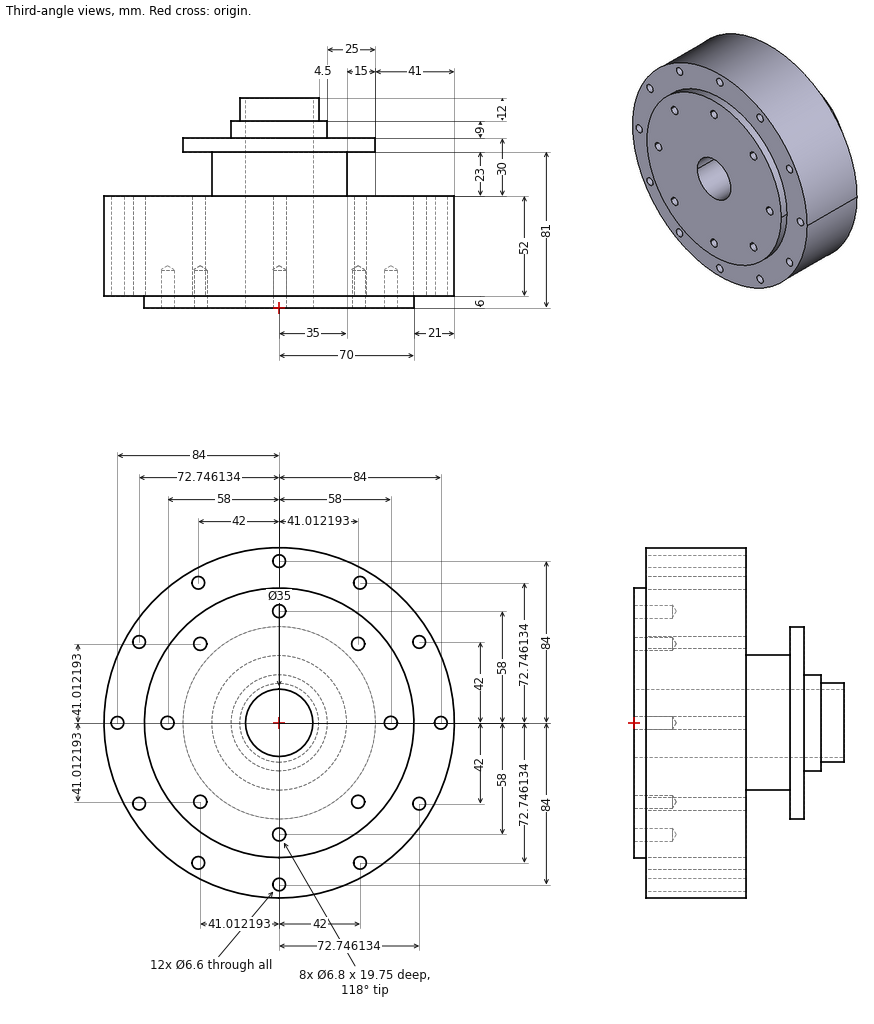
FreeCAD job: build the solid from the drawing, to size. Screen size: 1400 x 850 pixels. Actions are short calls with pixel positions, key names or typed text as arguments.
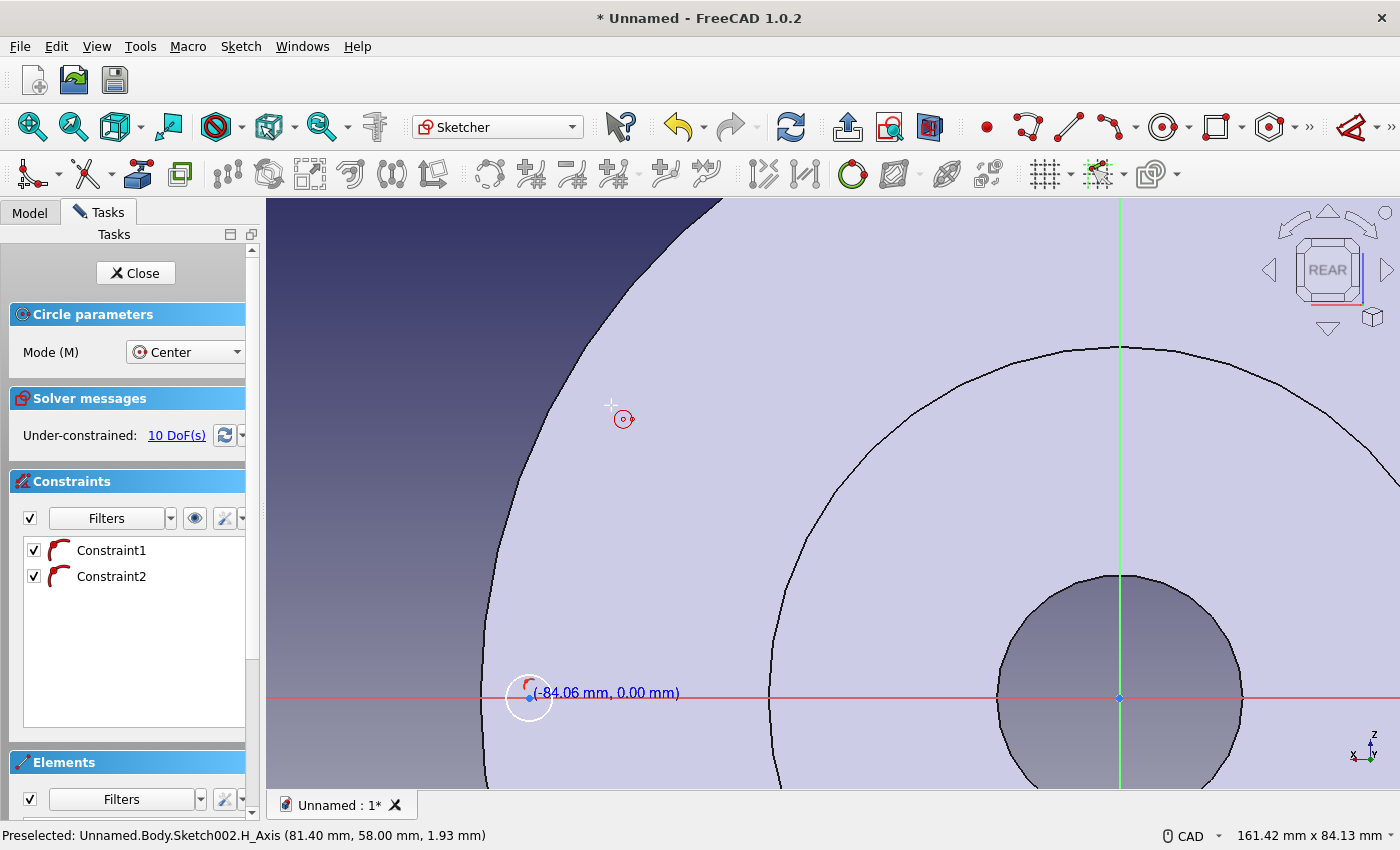
click(609, 403)
click(625, 387)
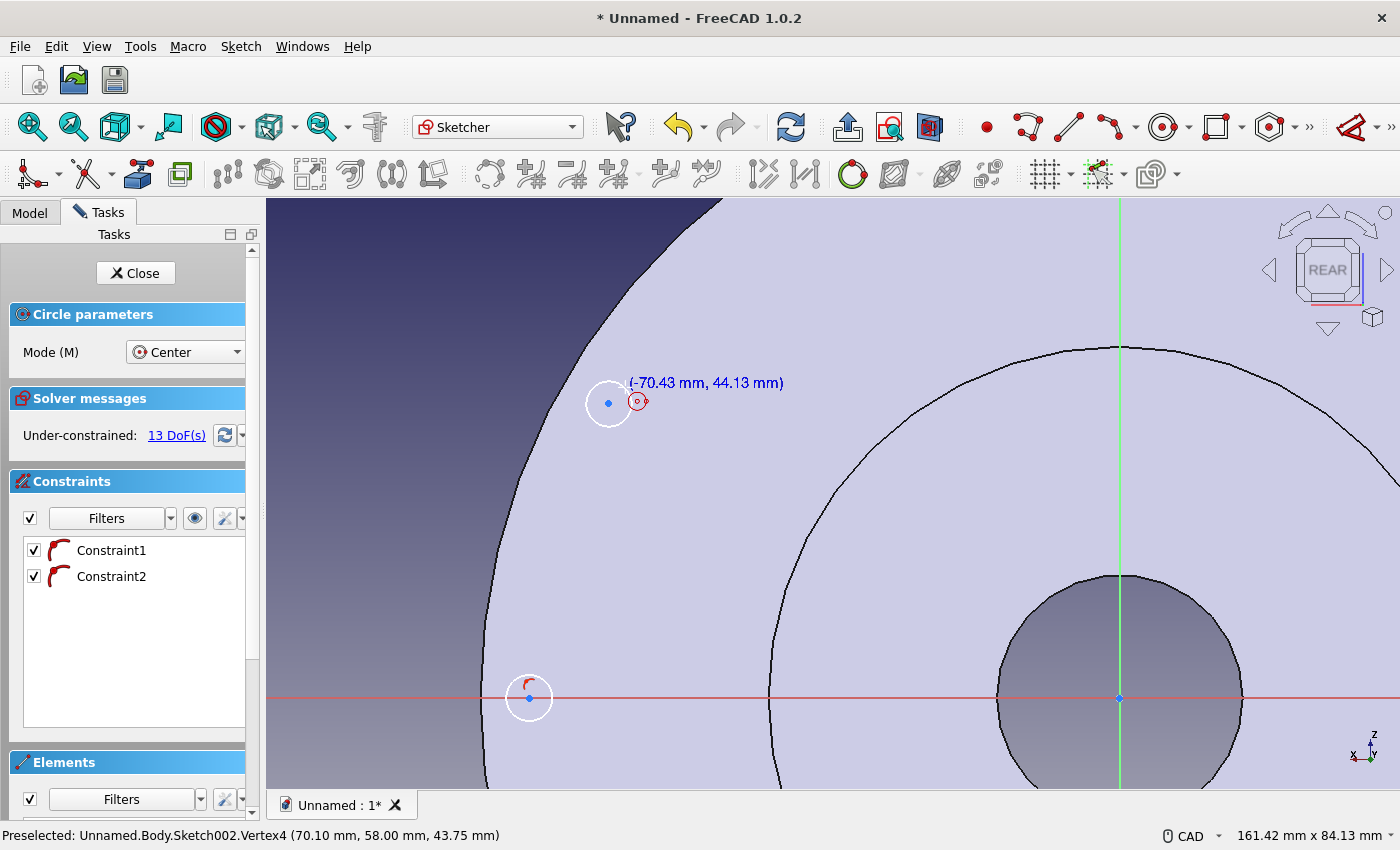
scroll(611, 405, down, 6)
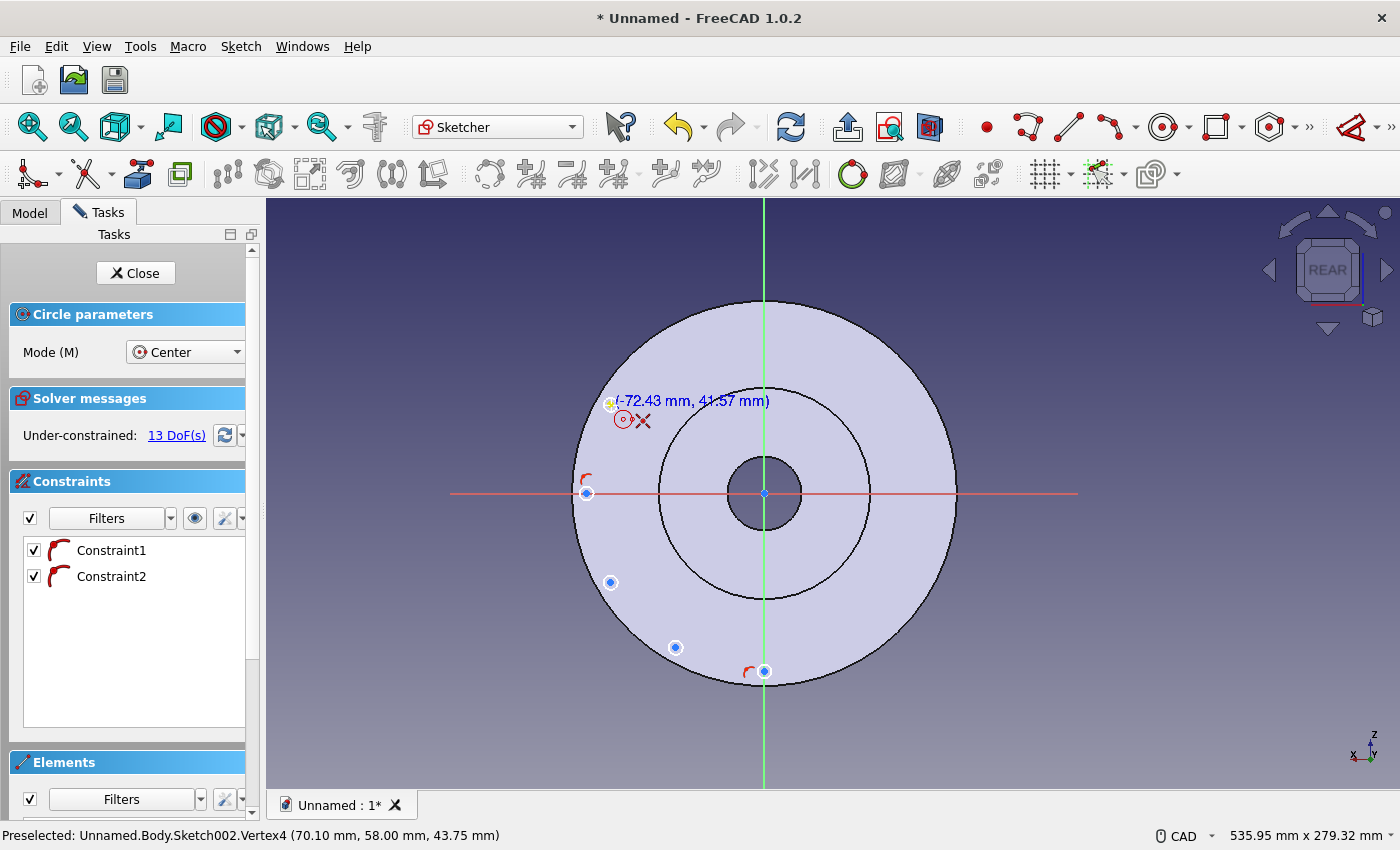
scroll(676, 340, up, 6)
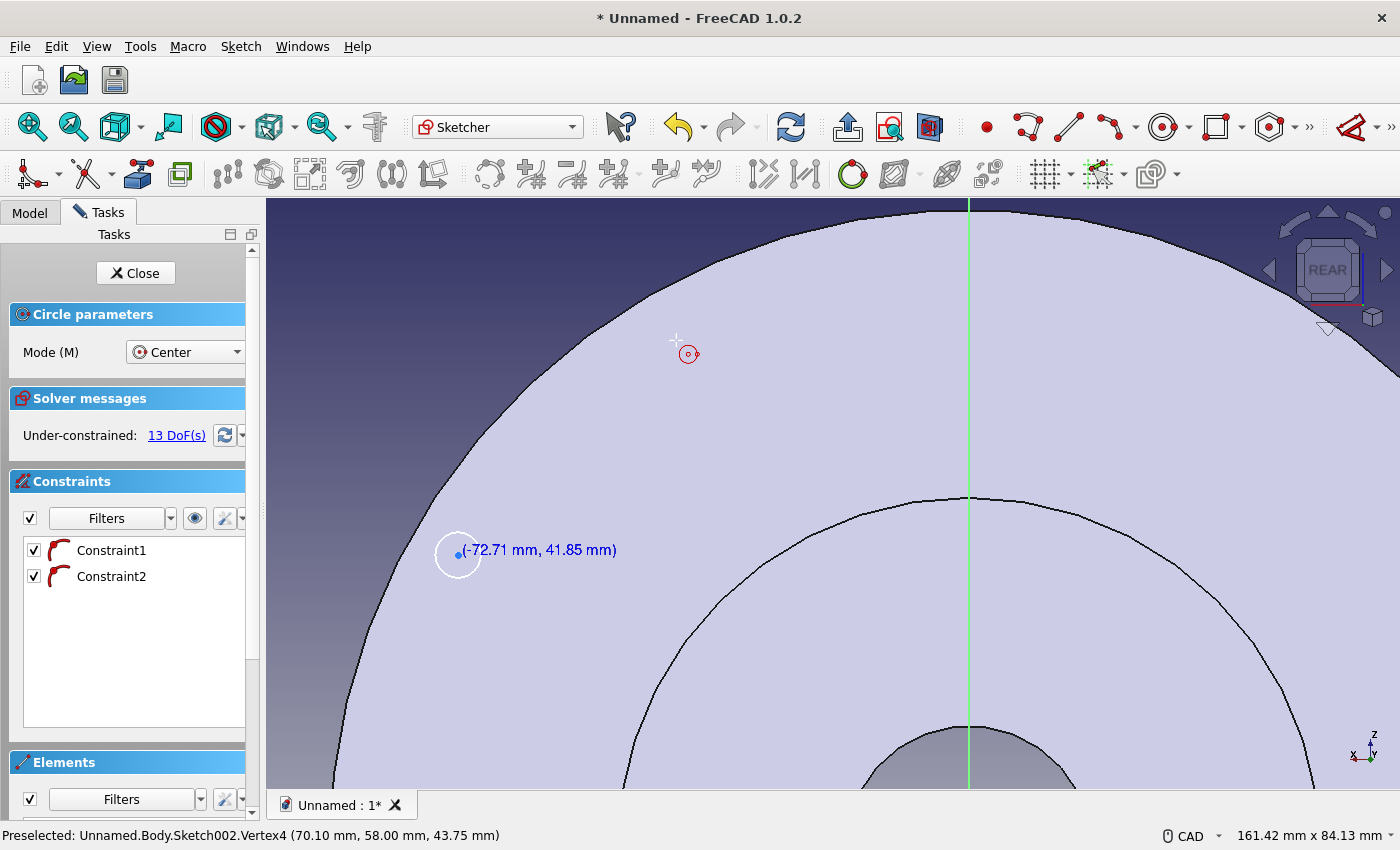
click(674, 338)
click(690, 322)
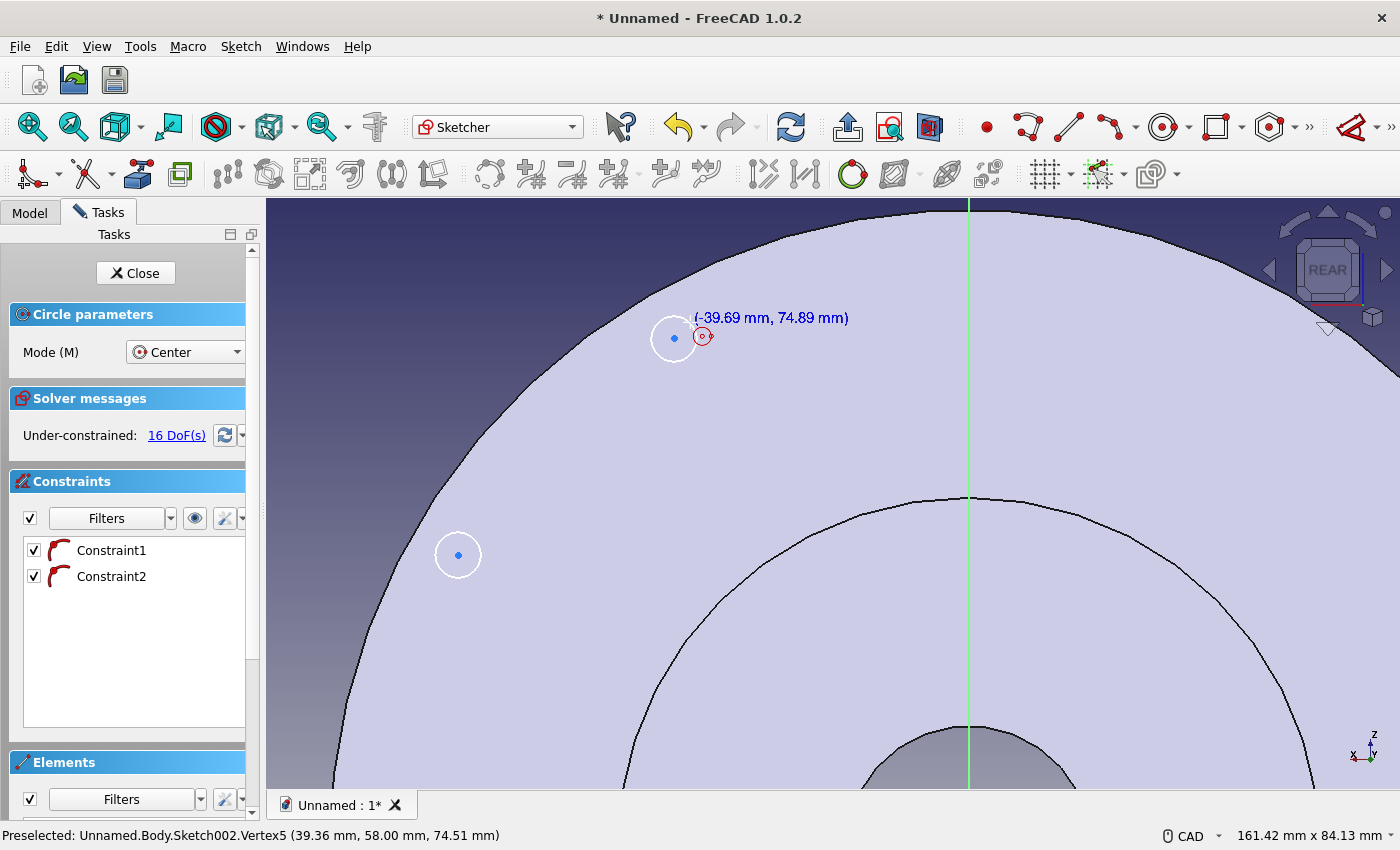
click(969, 259)
click(985, 243)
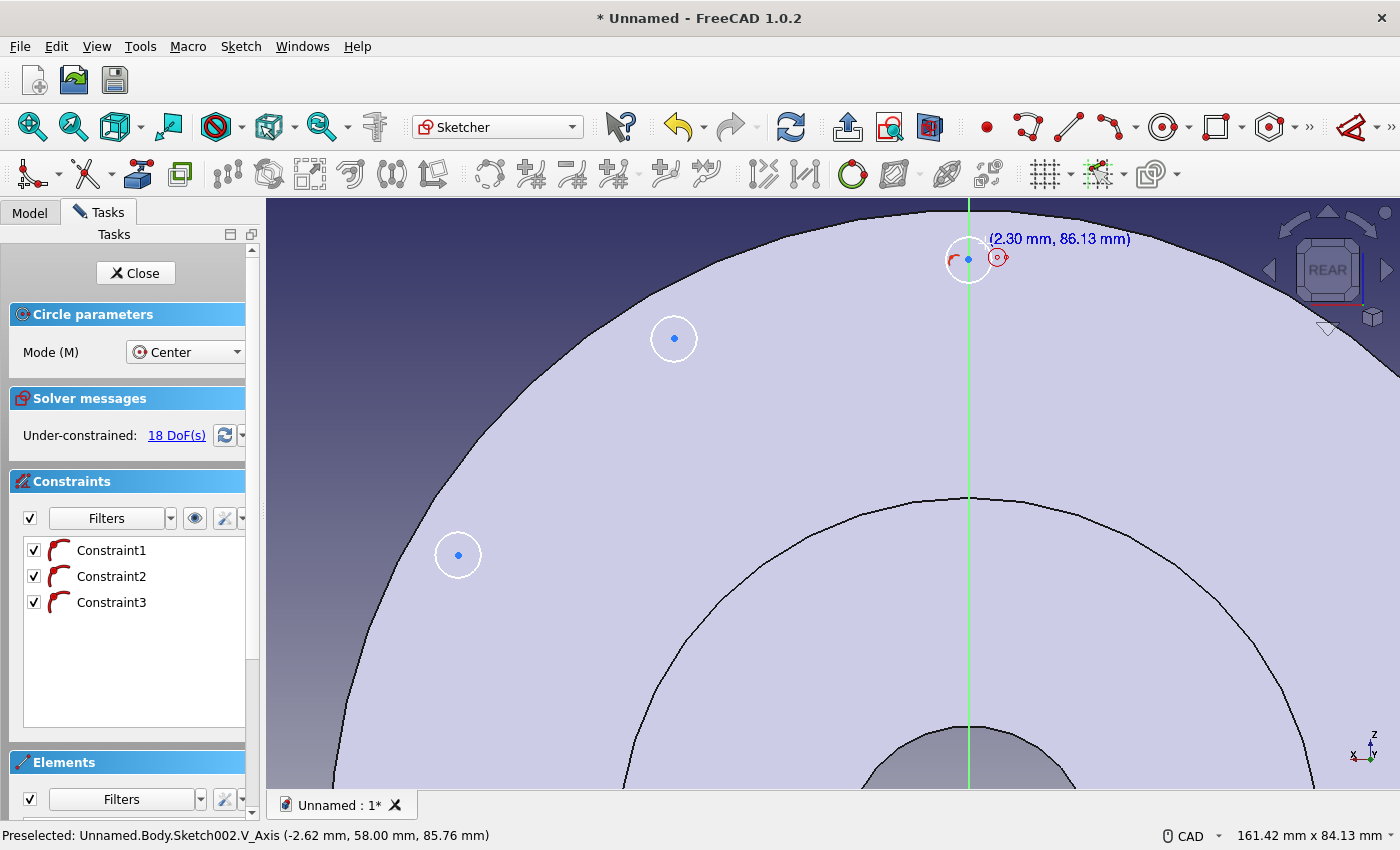
scroll(676, 340, down, 6)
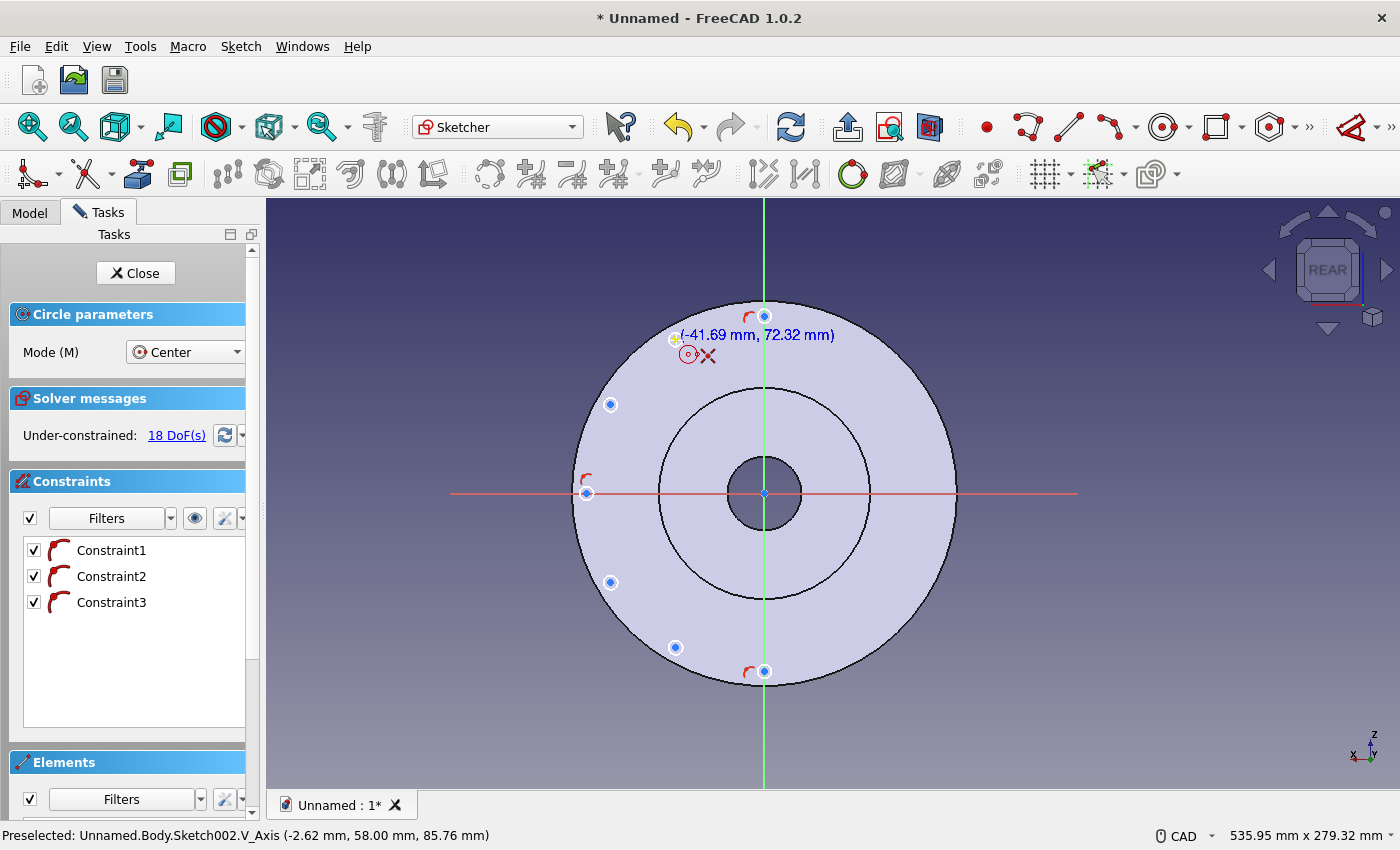
scroll(853, 340, up, 6)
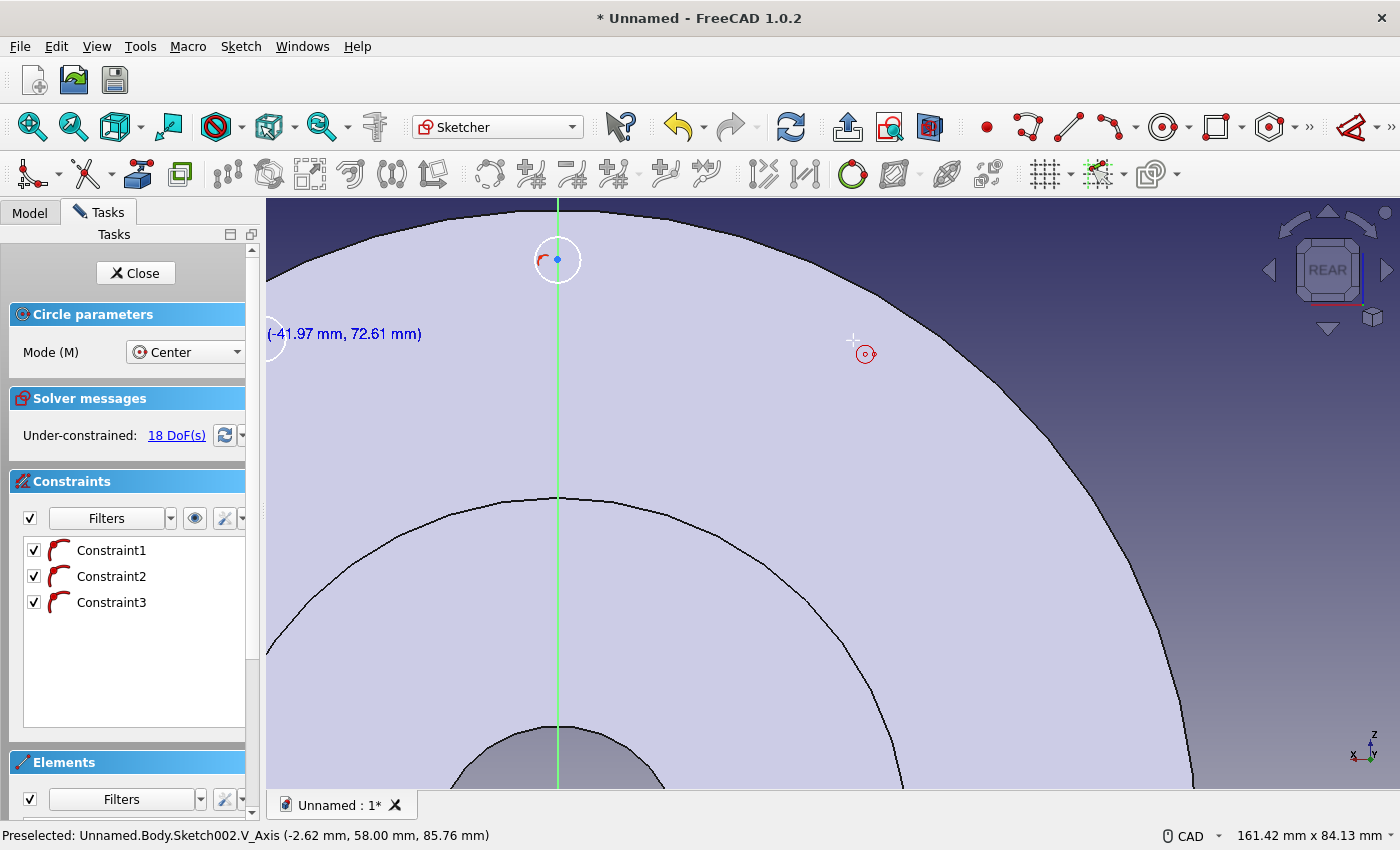
click(853, 338)
click(869, 322)